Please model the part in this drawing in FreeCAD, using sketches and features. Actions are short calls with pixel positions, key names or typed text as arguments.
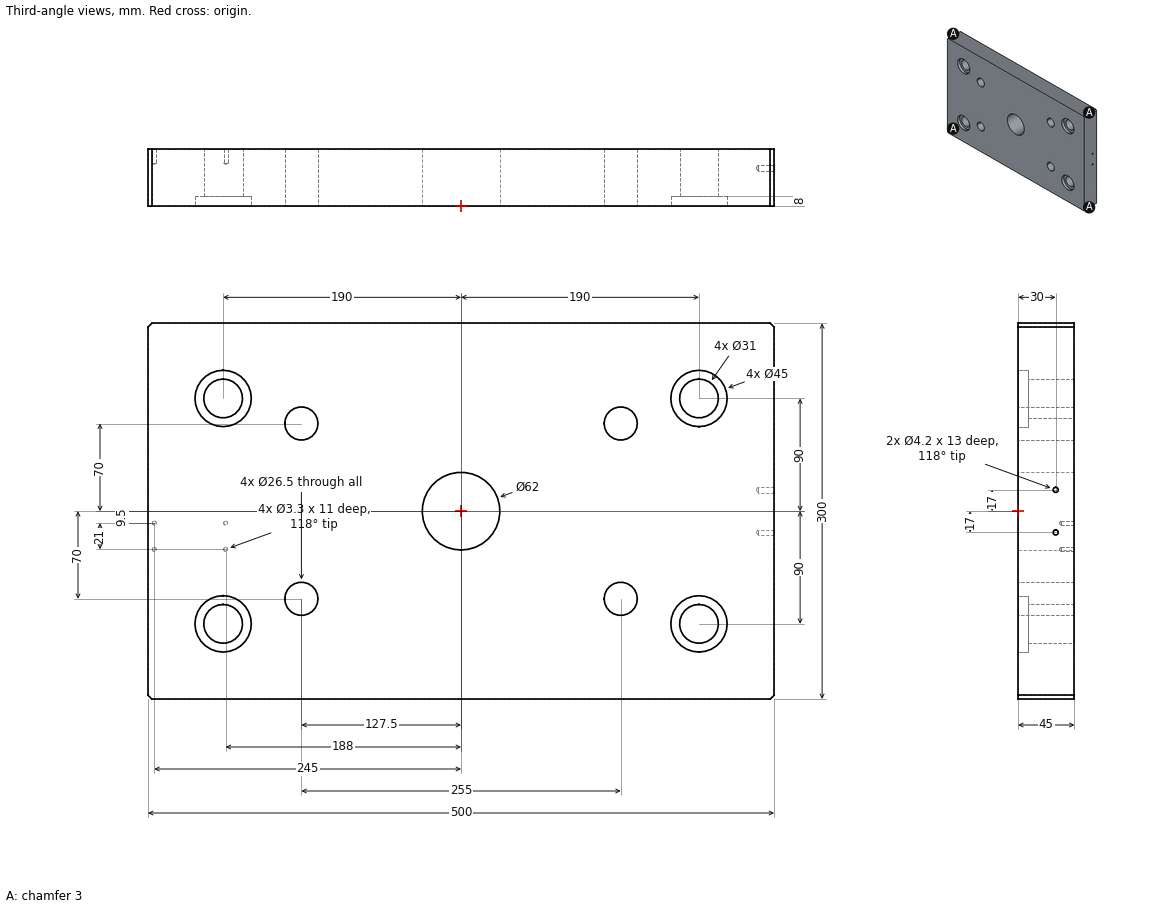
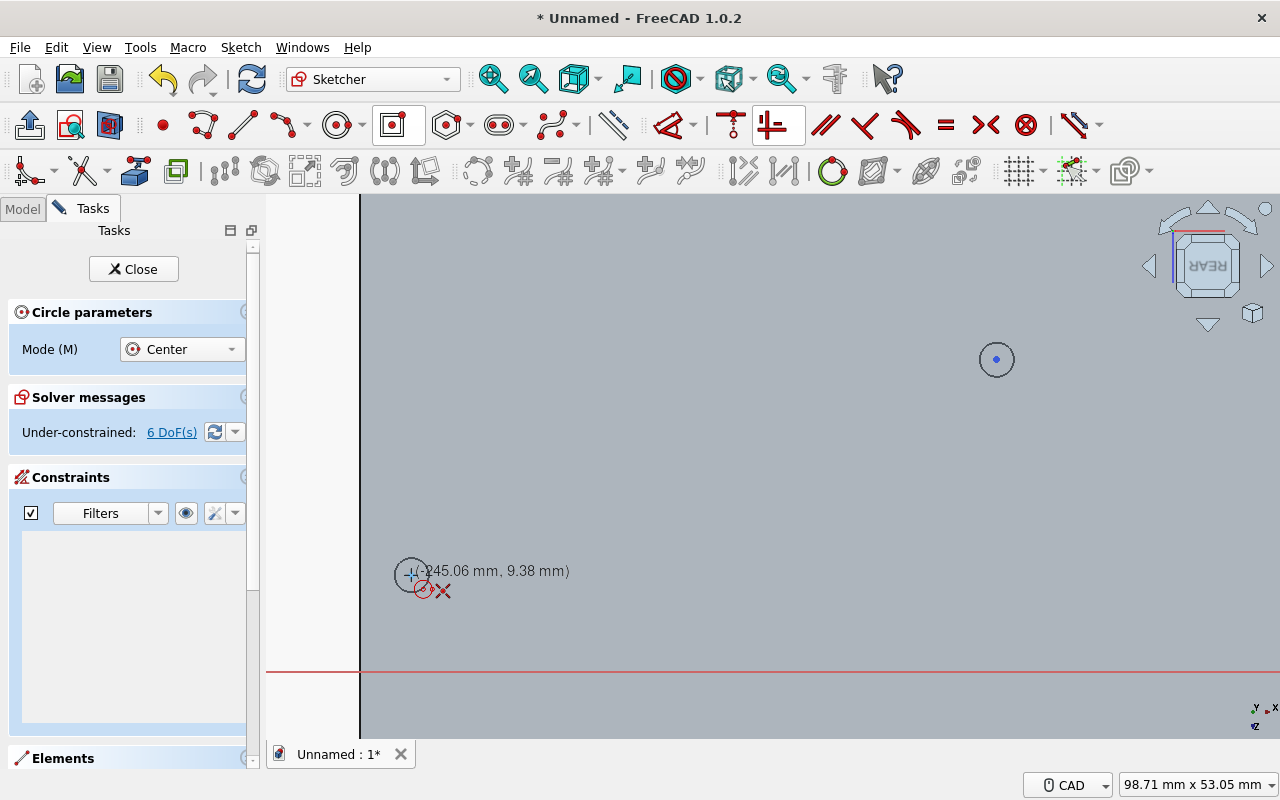
scroll(997, 575, up, 2)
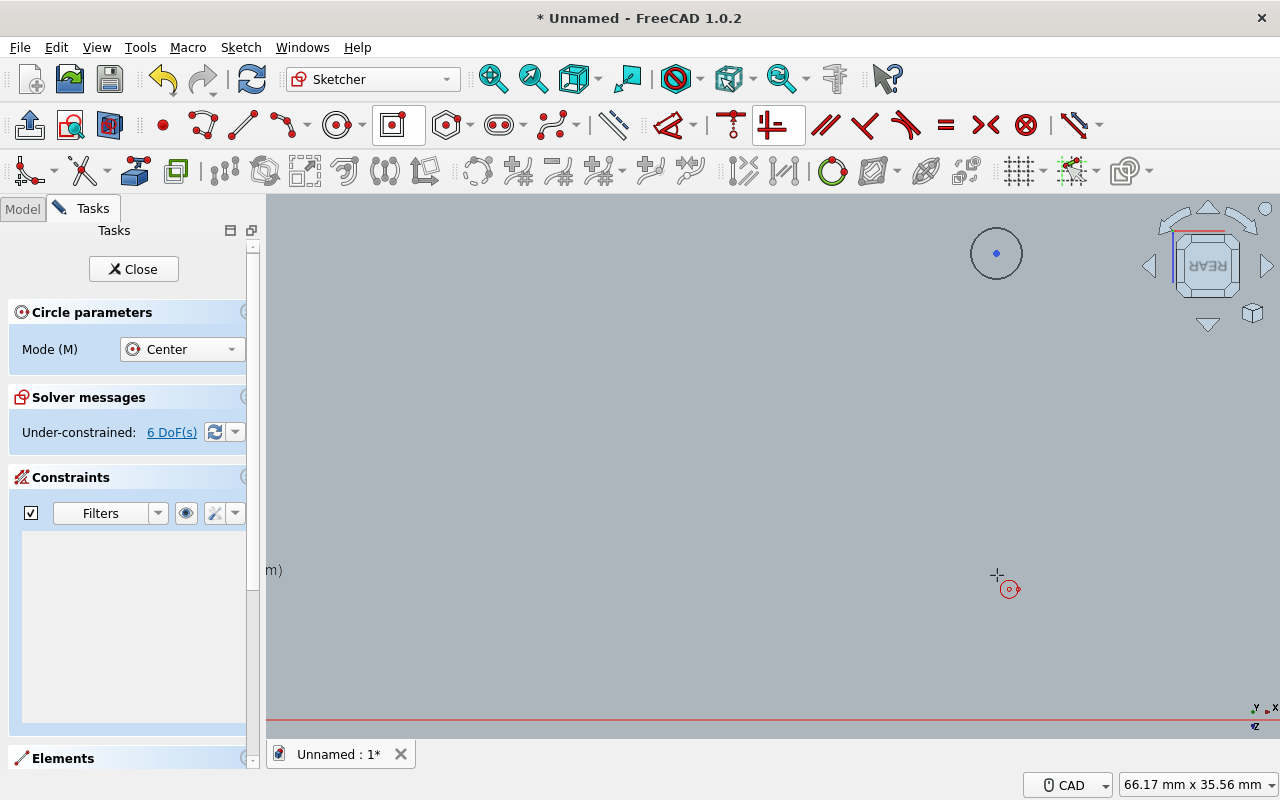
click(997, 574)
click(1015, 556)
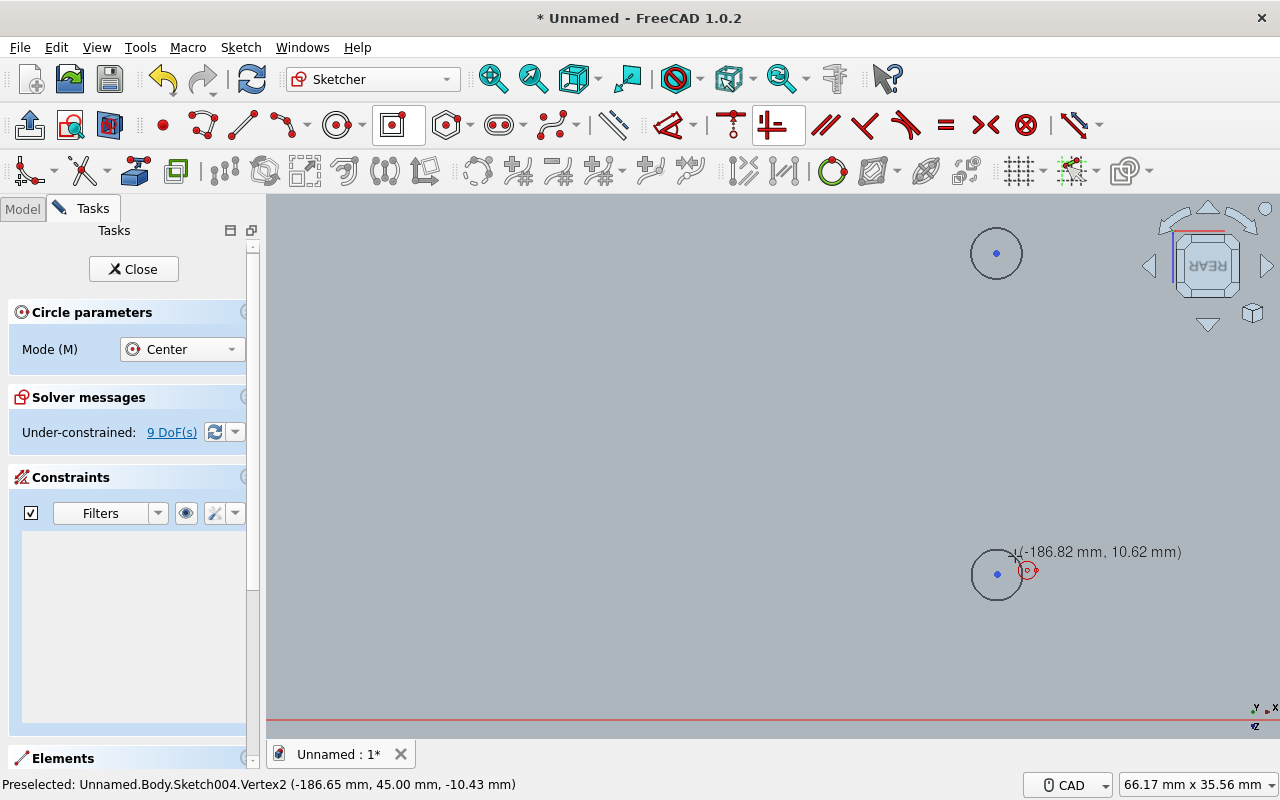
scroll(998, 575, down, 2)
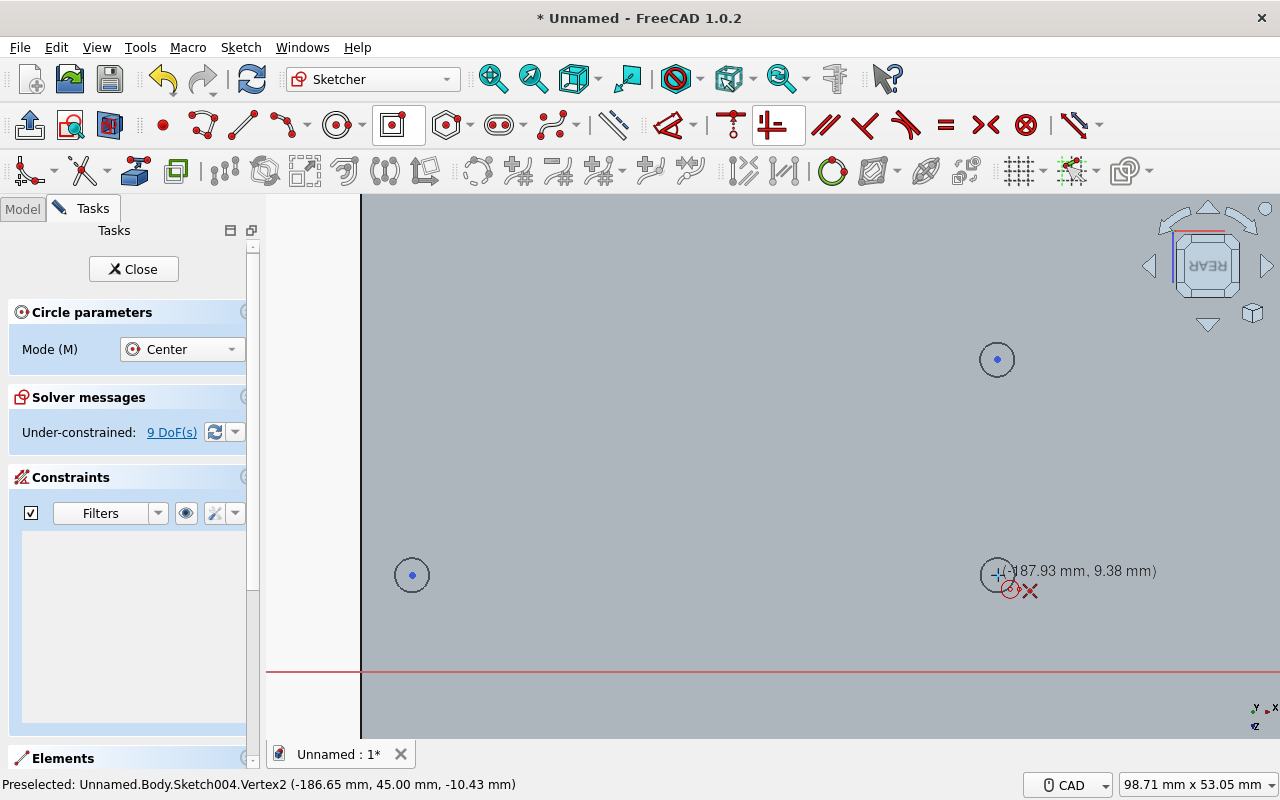
scroll(412, 359, up, 2)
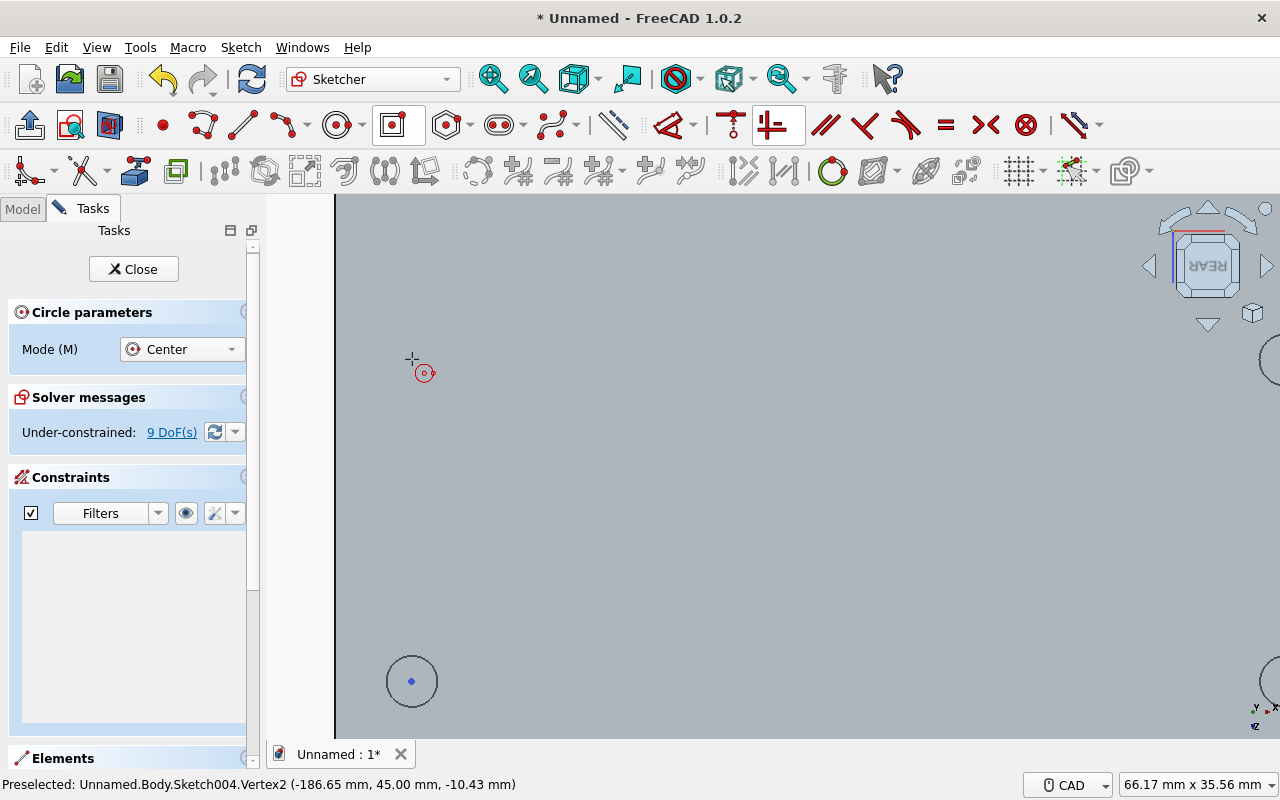
click(412, 359)
click(430, 341)
key(Escape)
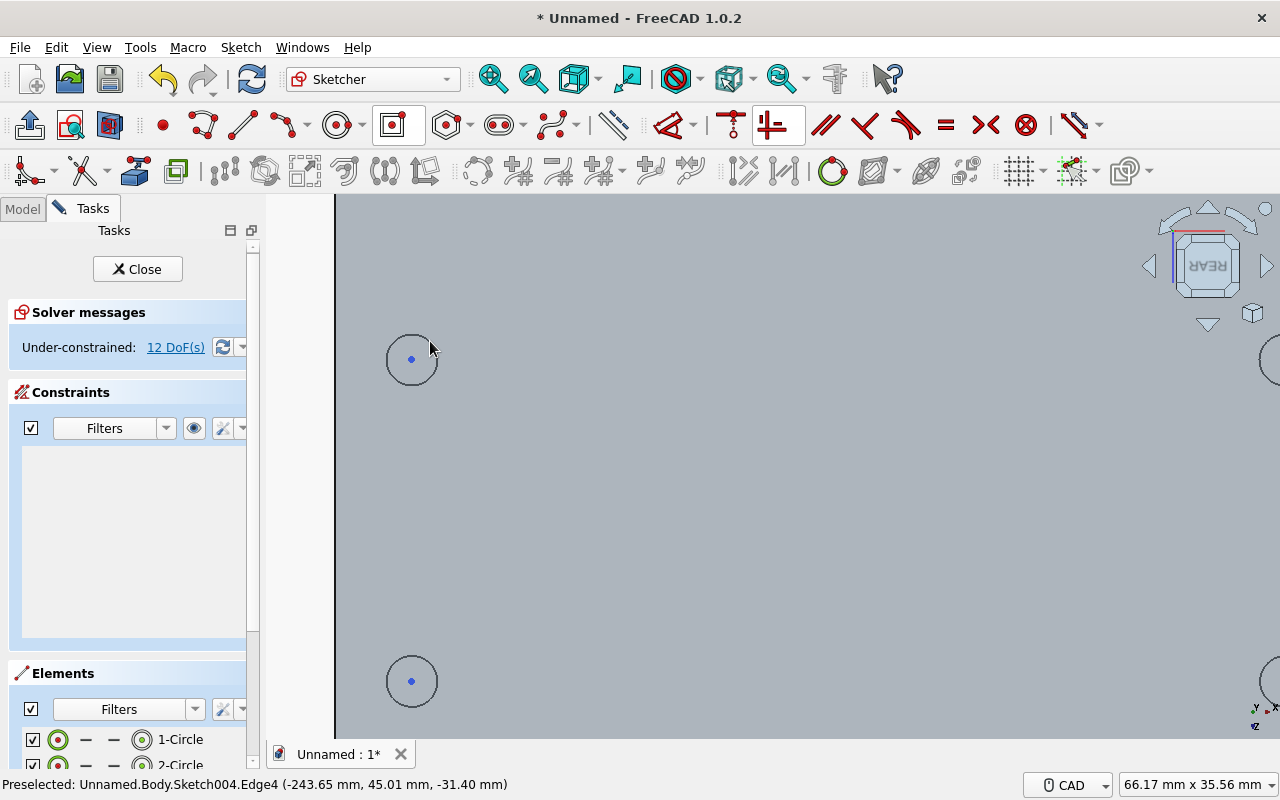
scroll(411, 358, down, 2)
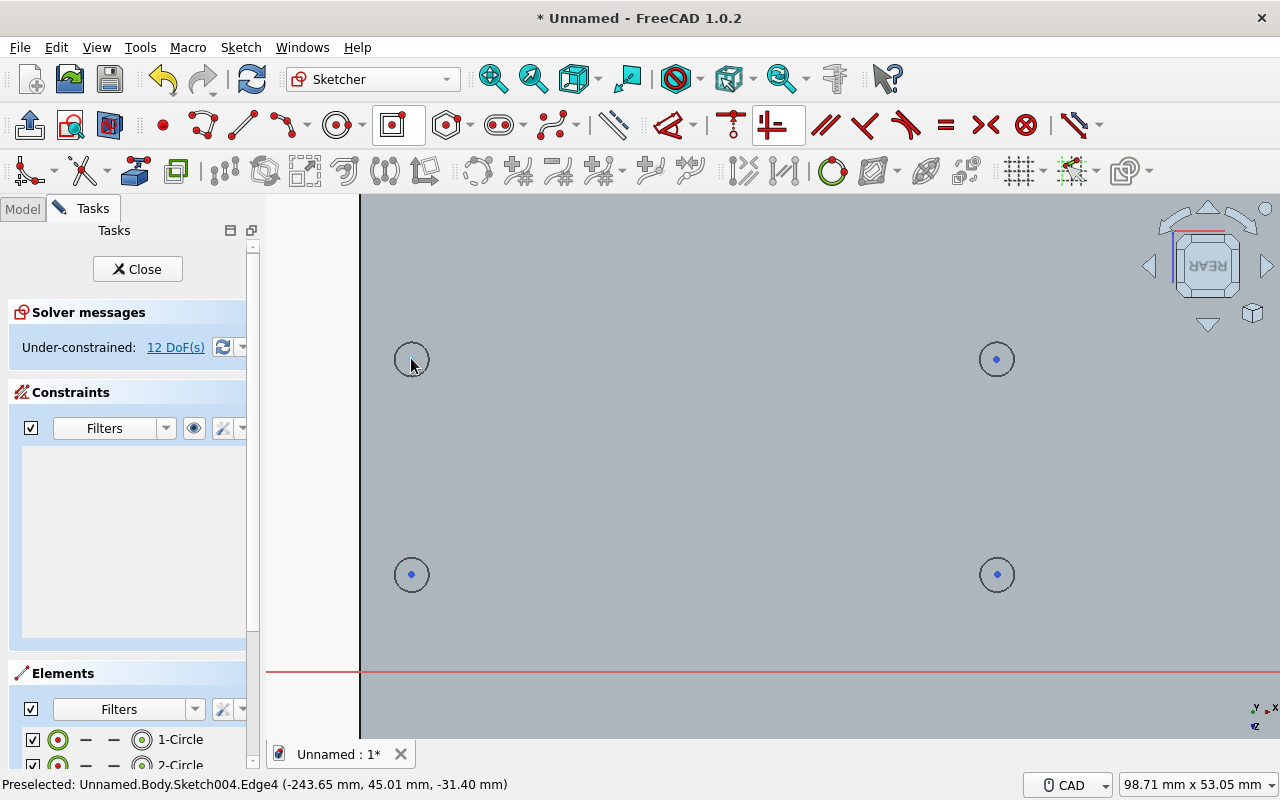
click(1009, 347)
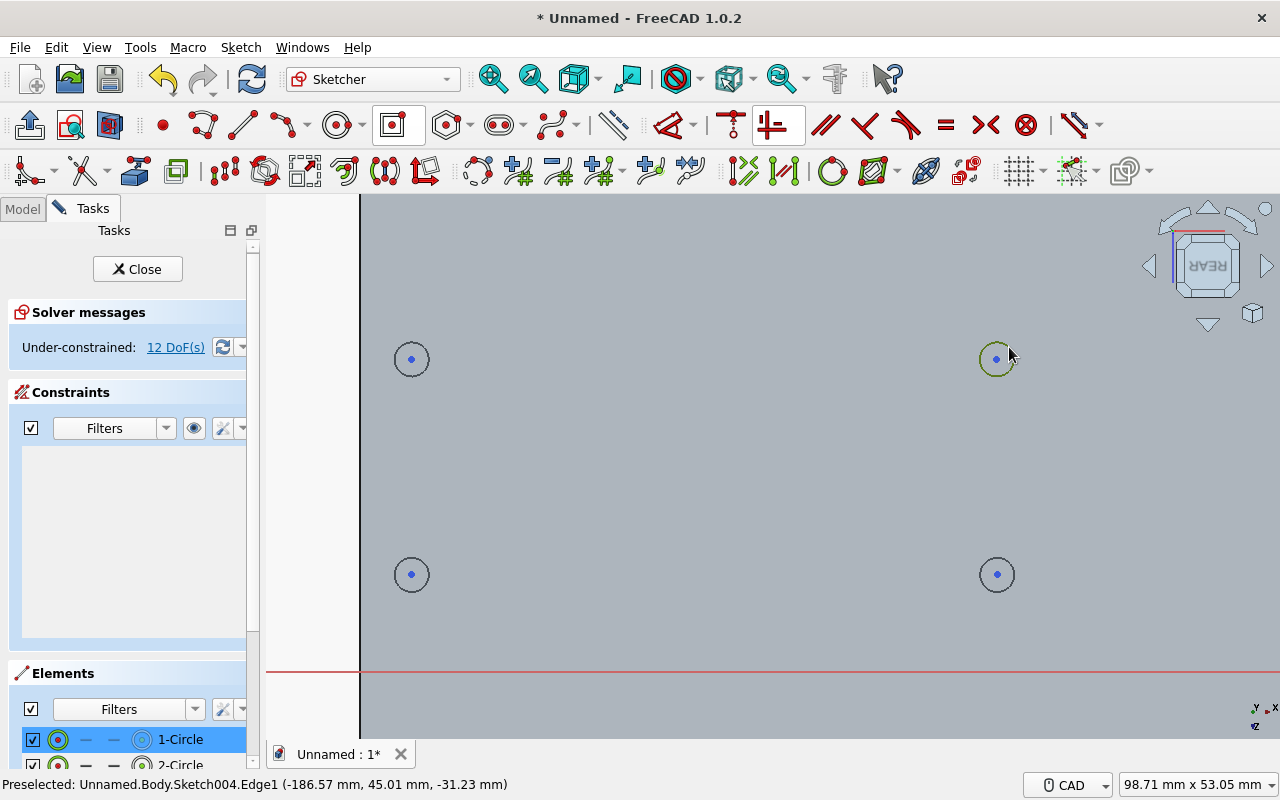
click(424, 563)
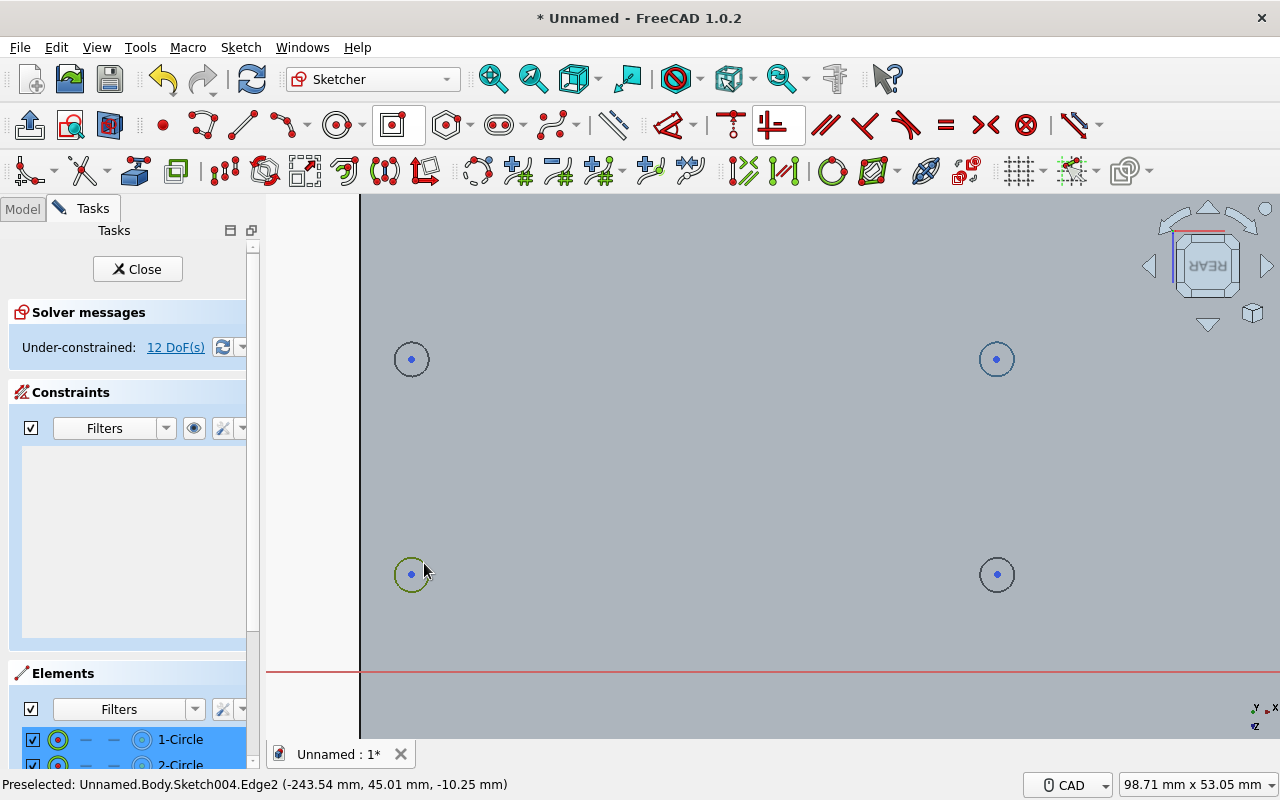
click(1009, 563)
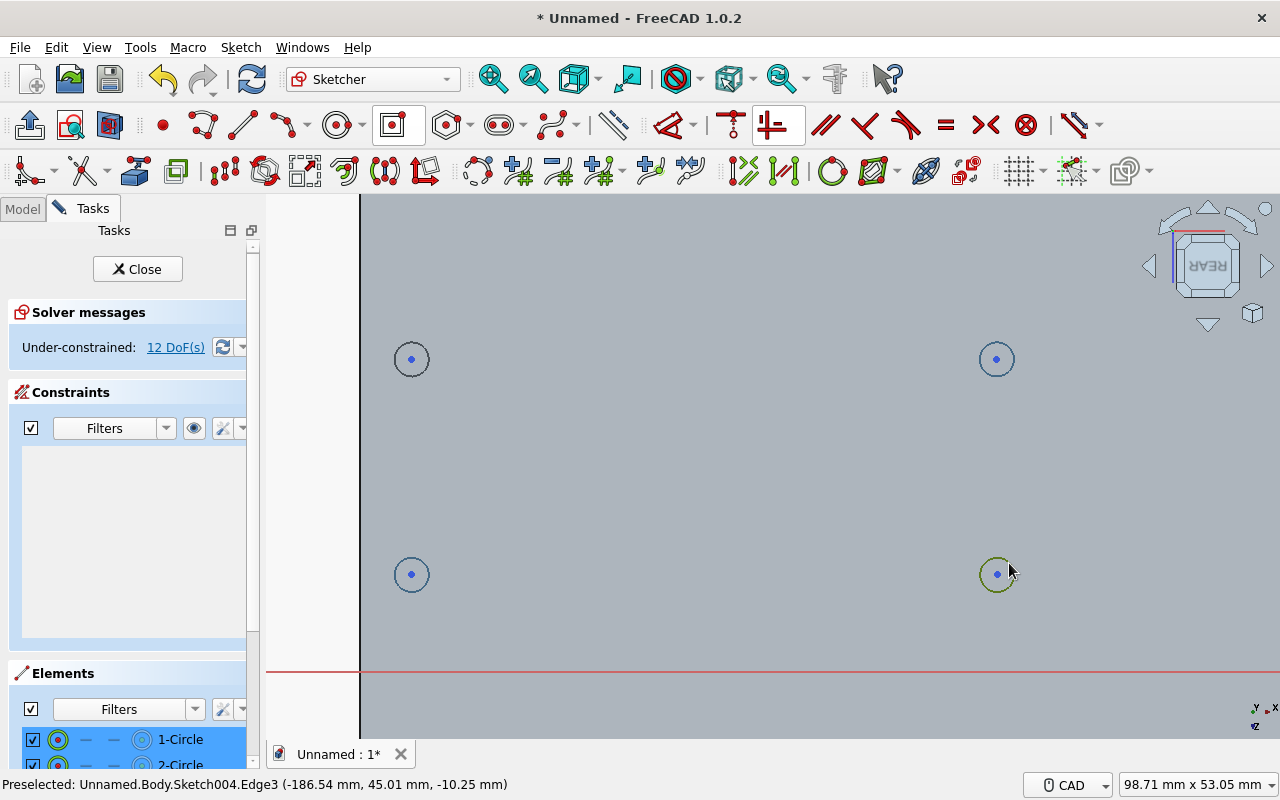
click(424, 347)